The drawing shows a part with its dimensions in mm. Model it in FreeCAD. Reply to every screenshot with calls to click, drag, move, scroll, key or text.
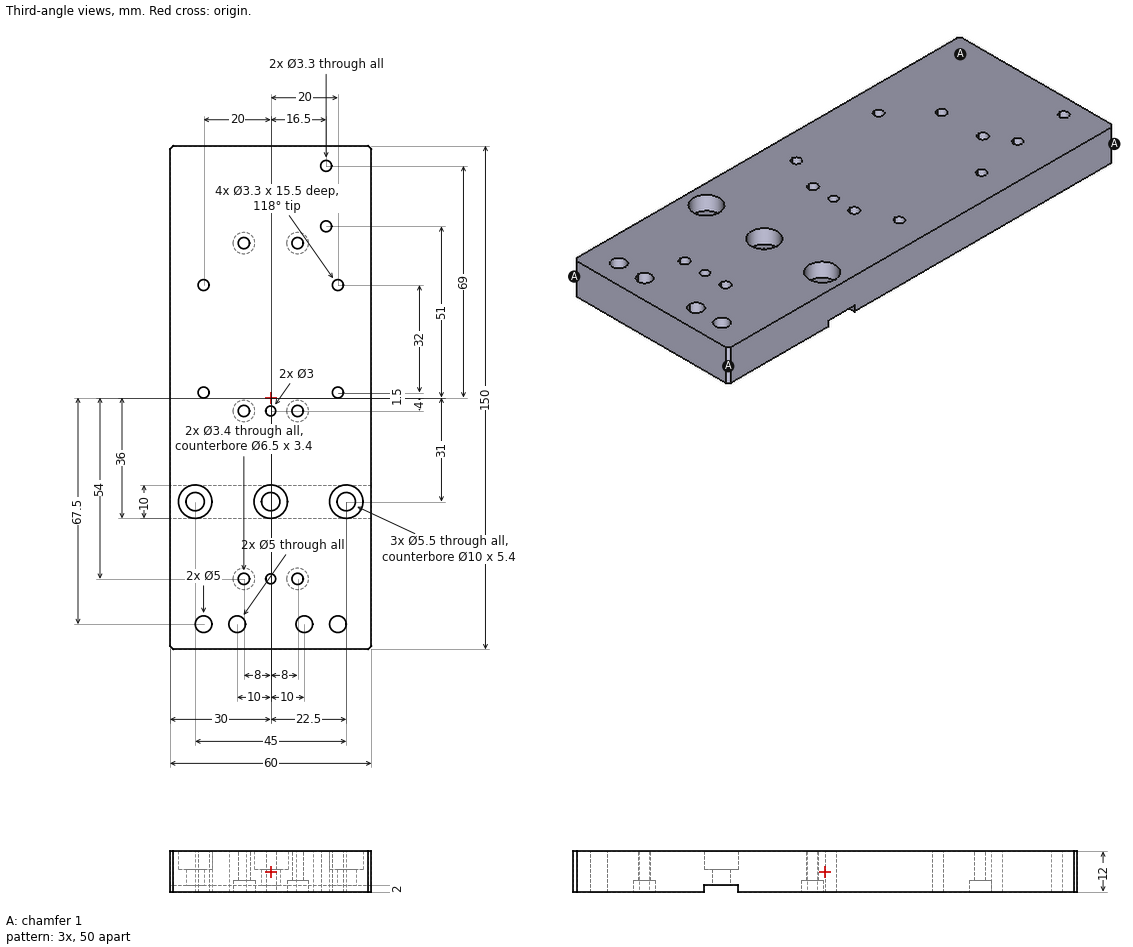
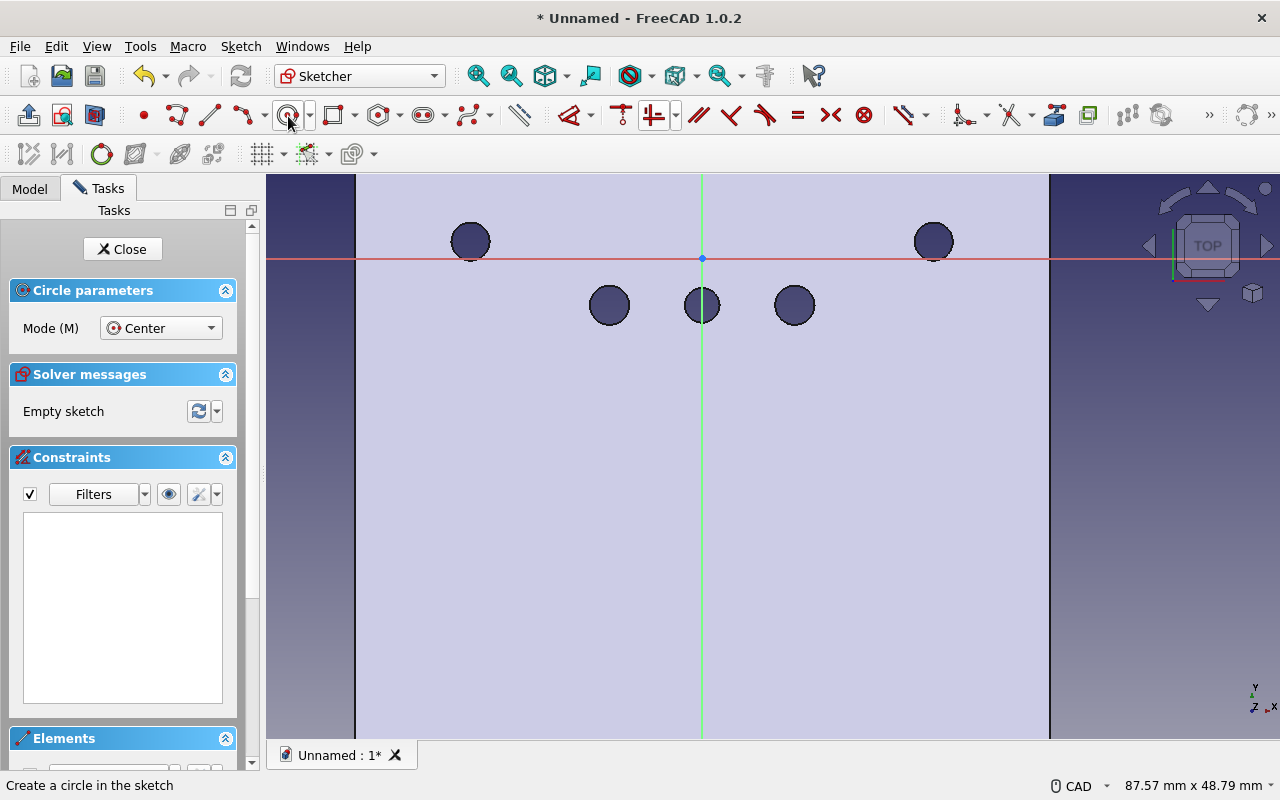
click(963, 618)
click(985, 595)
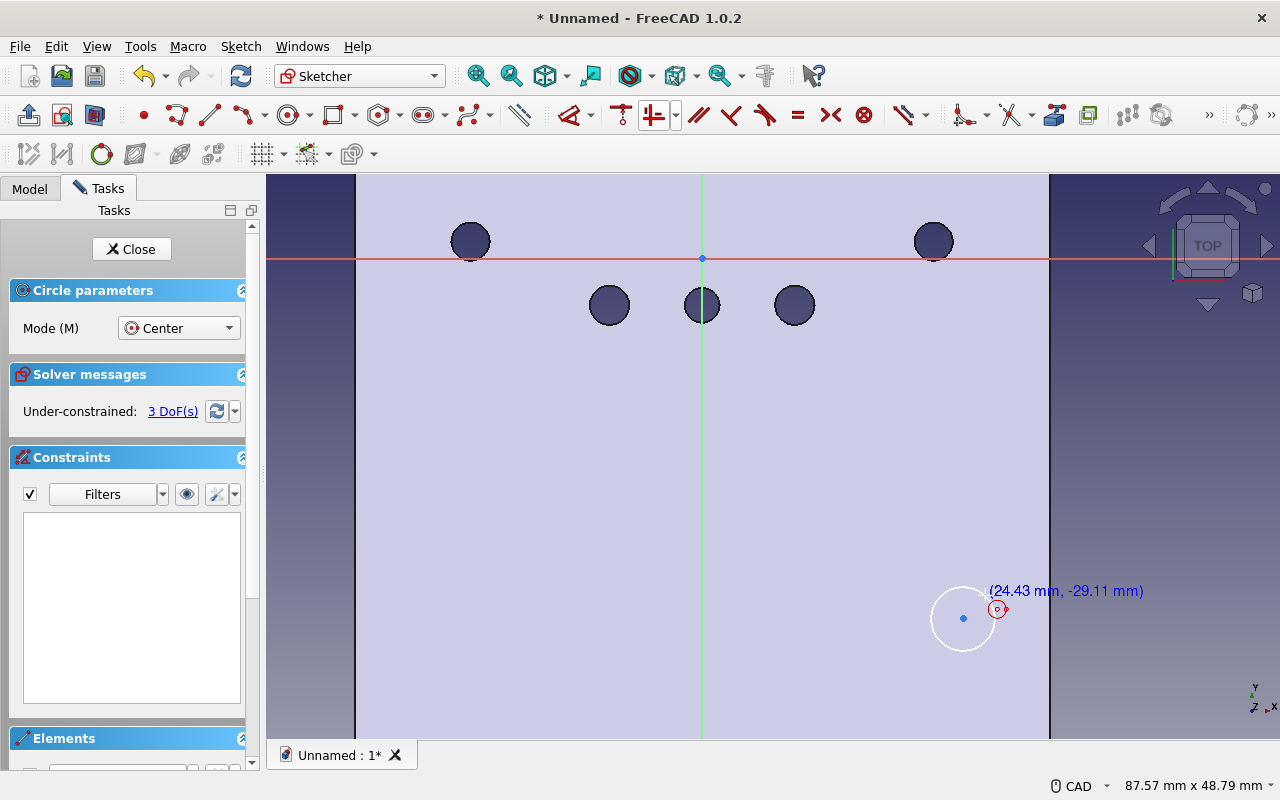
click(702, 618)
click(725, 595)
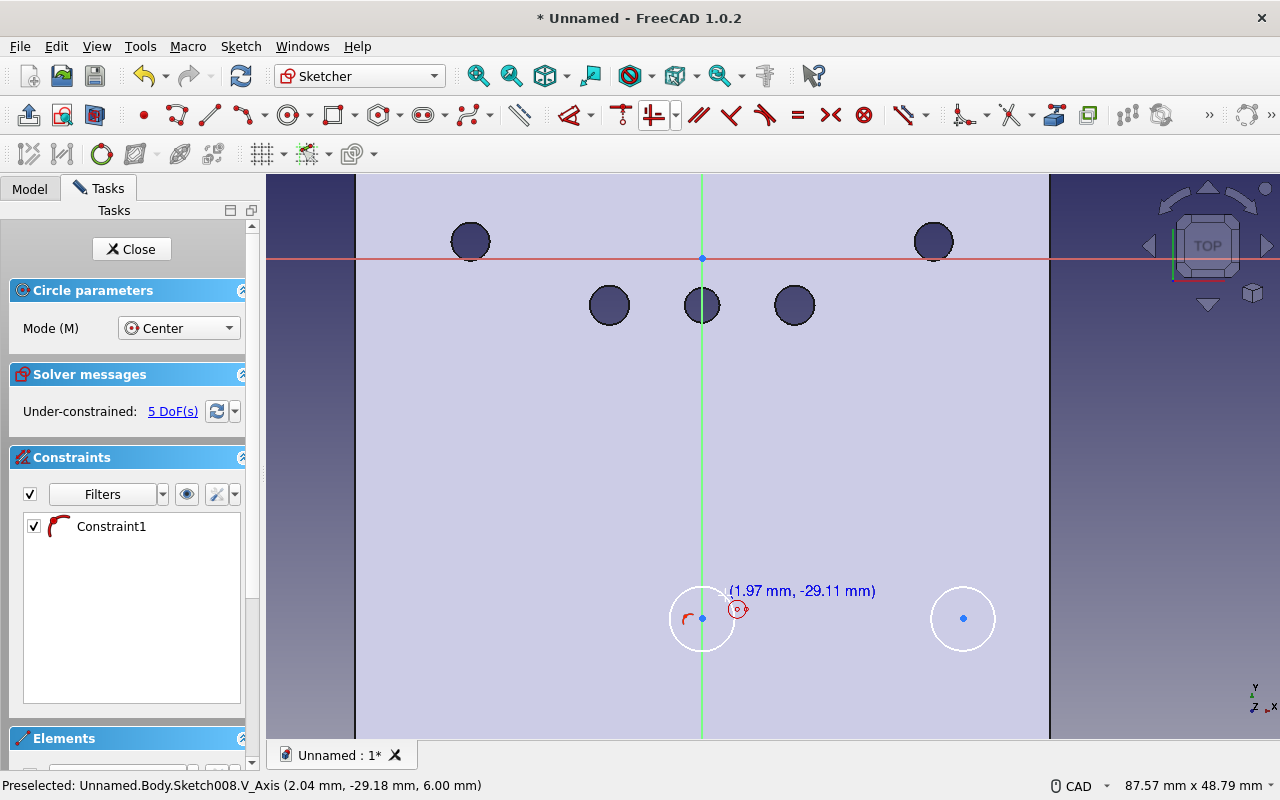
click(442, 618)
click(464, 595)
key(Escape)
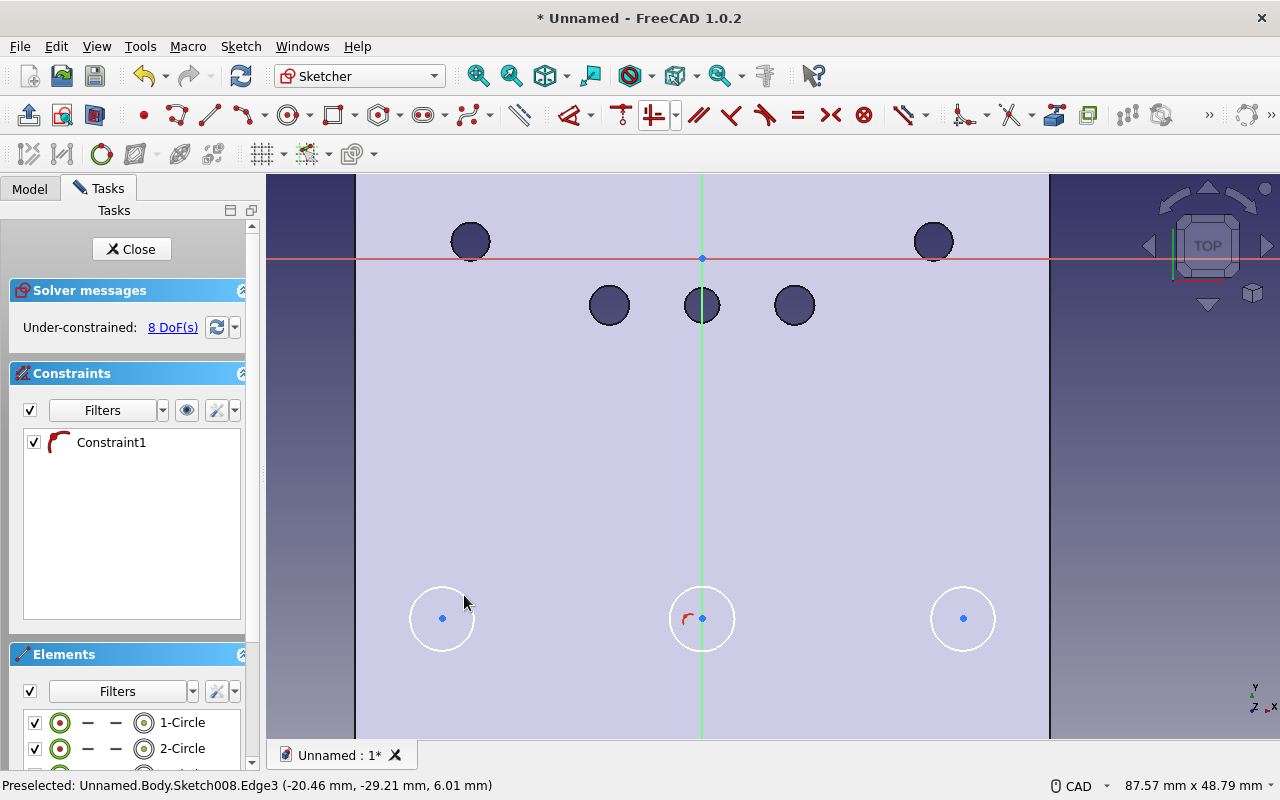
click(985, 596)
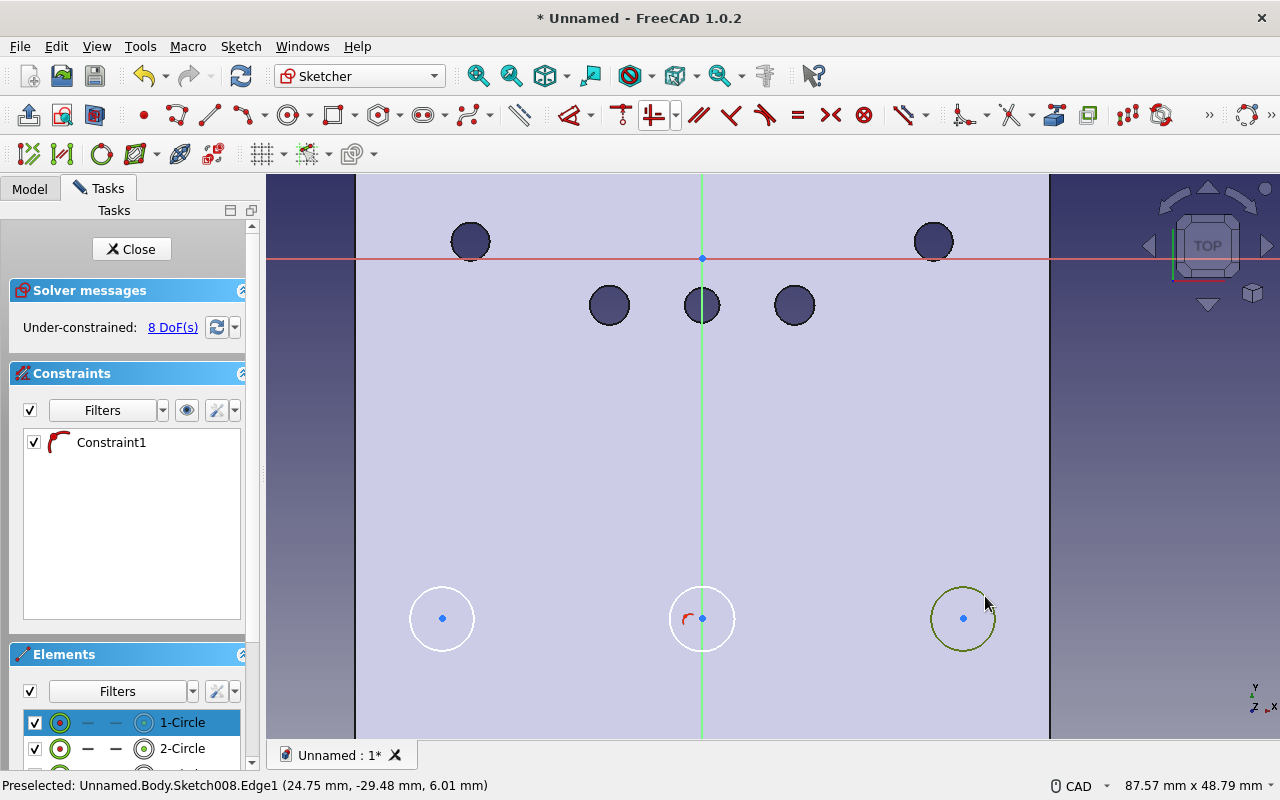
click(725, 596)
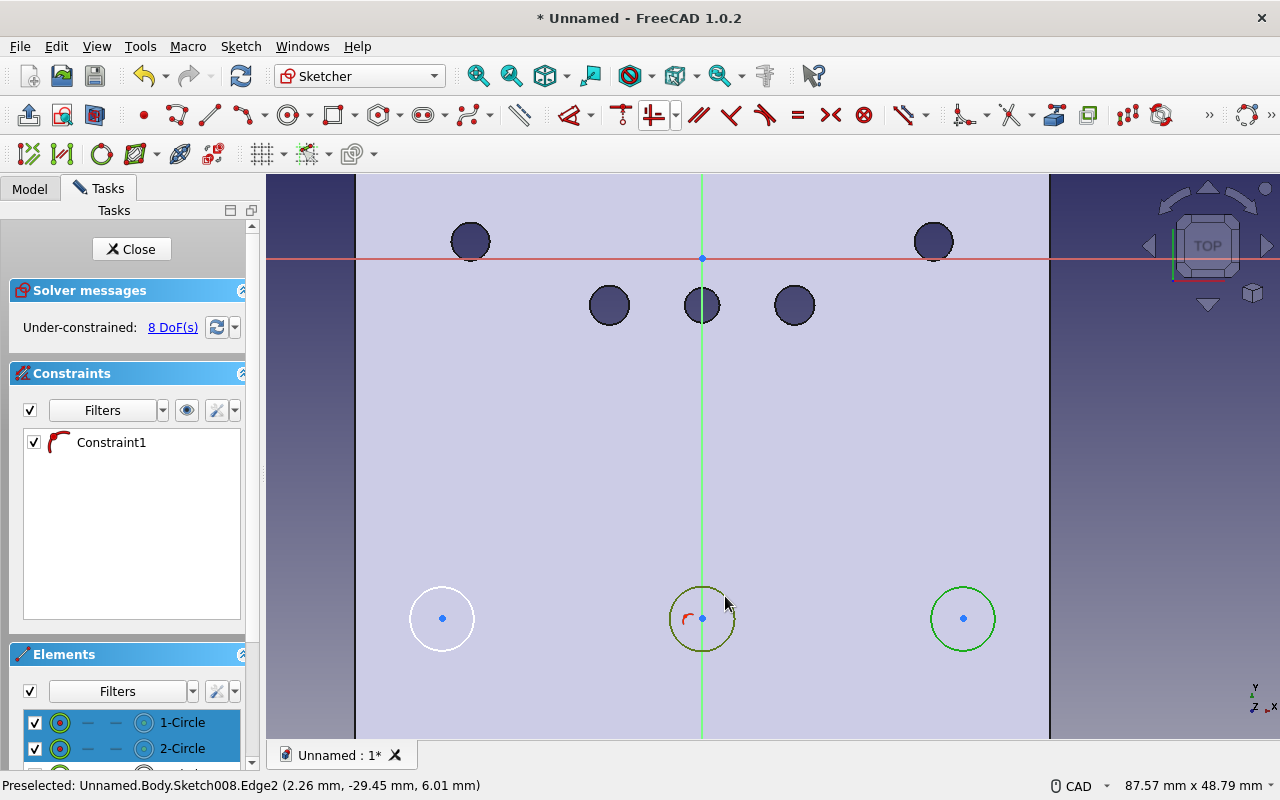
click(464, 596)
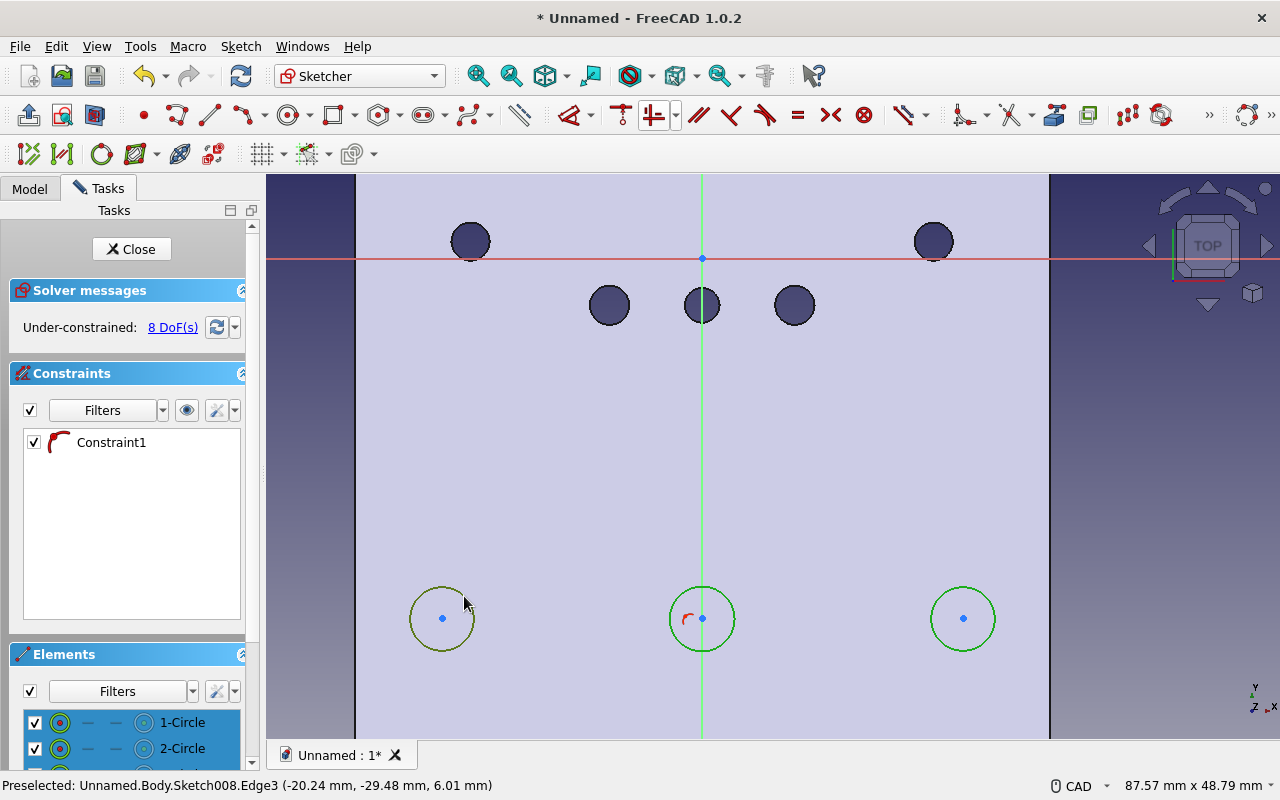
click(798, 116)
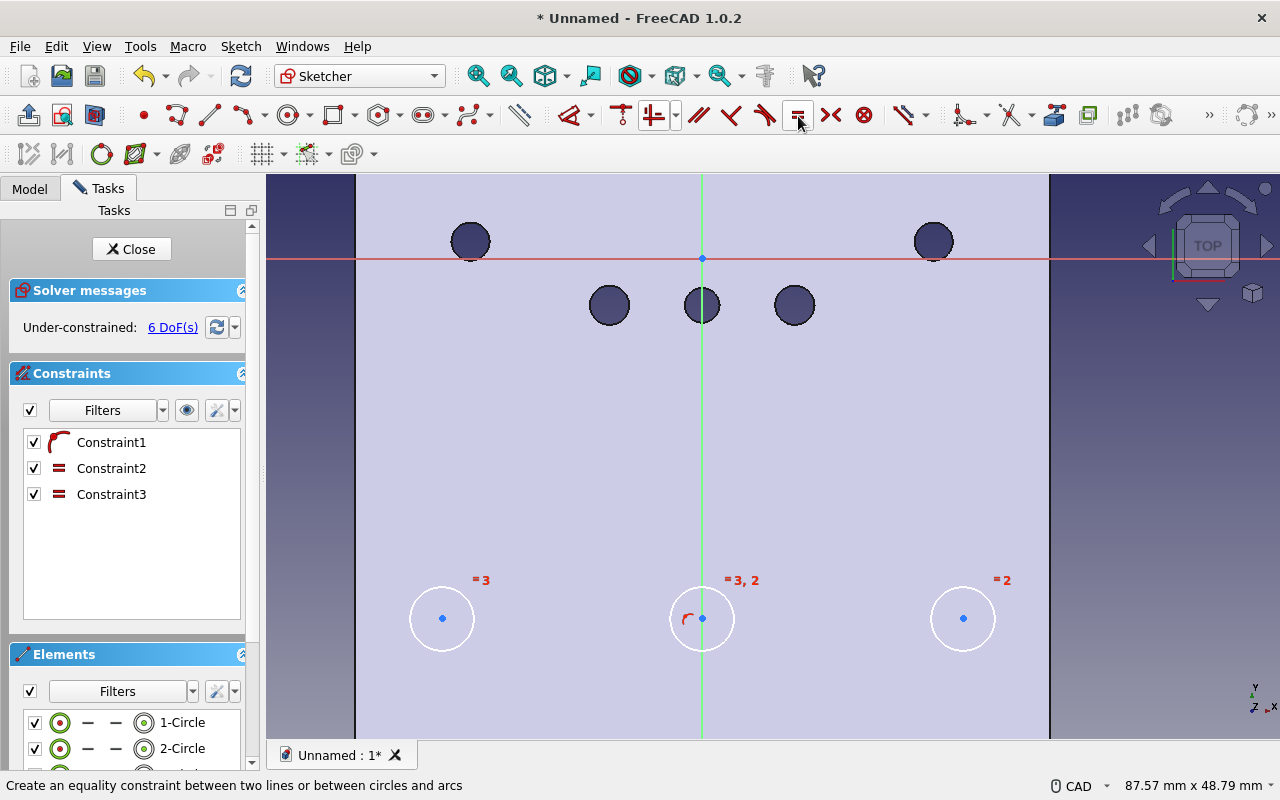
click(963, 619)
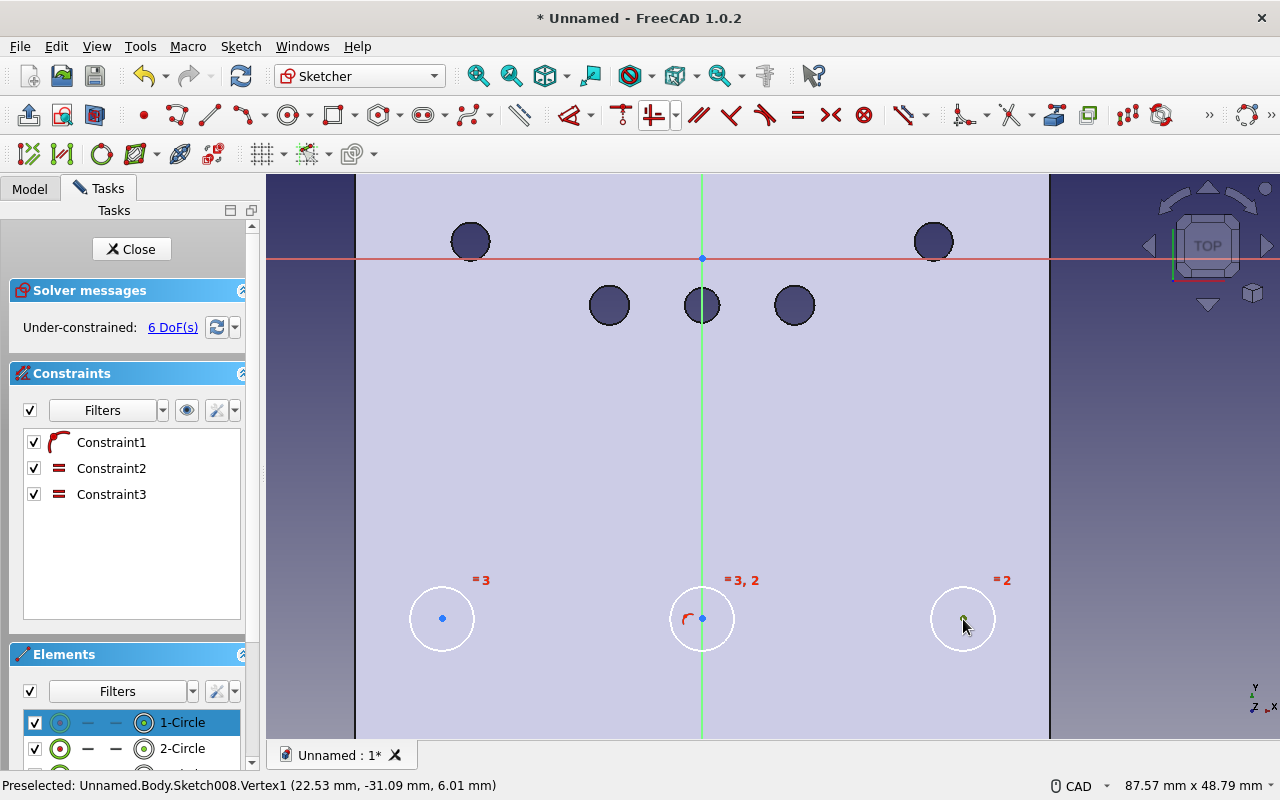
click(702, 619)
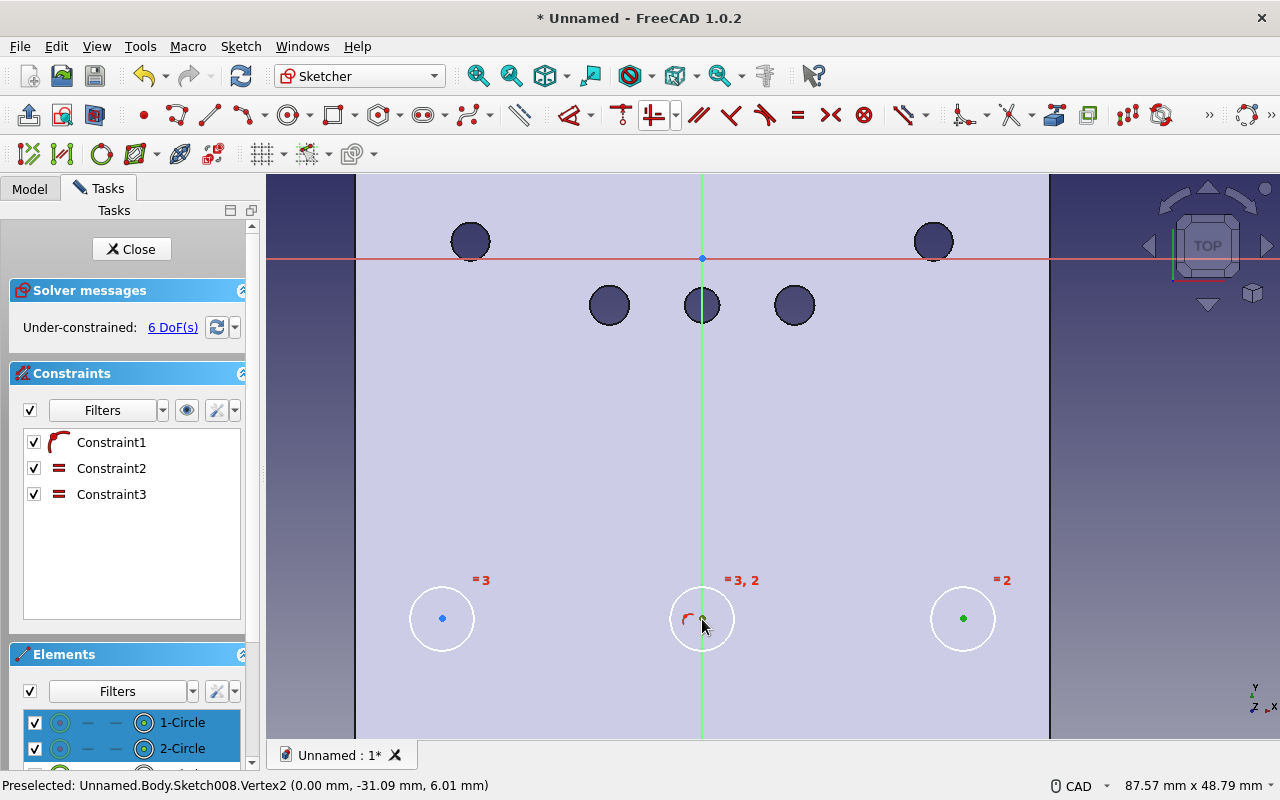
key(h)